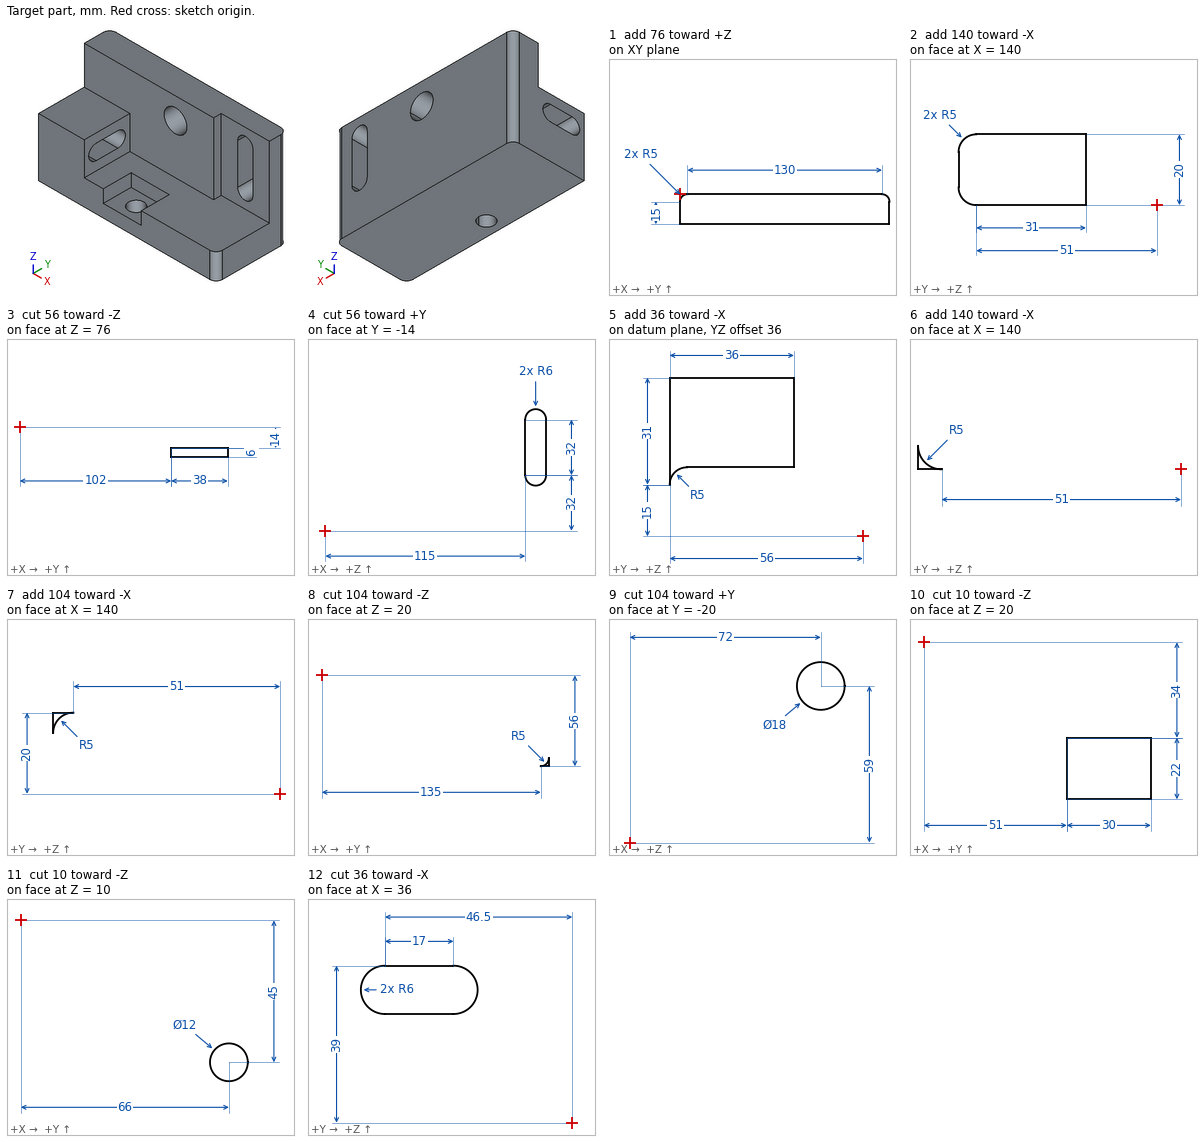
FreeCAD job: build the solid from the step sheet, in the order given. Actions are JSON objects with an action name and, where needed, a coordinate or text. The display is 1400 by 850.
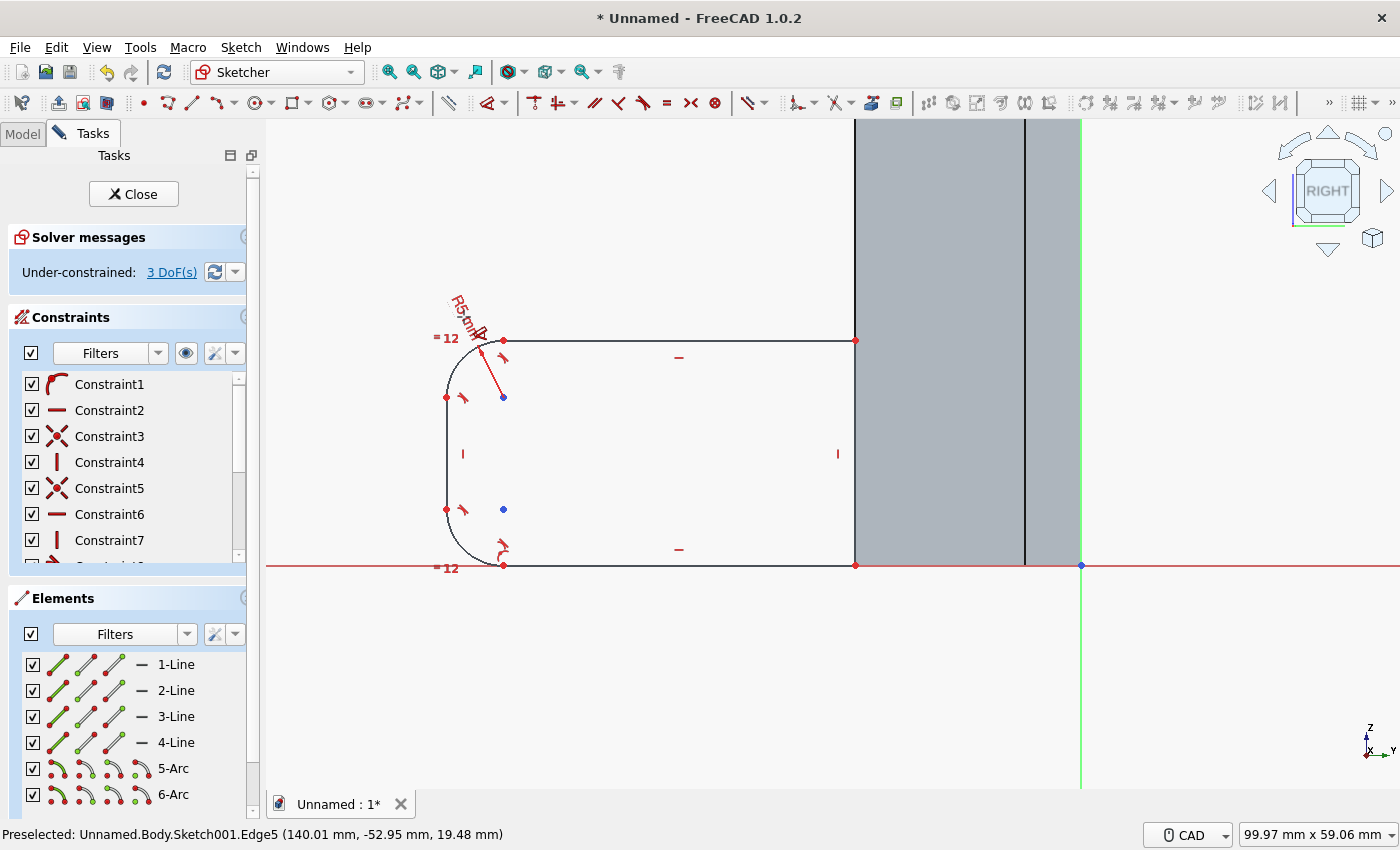
{"action": "left_click", "coordinate": [609, 566]}
{"action": "left_click", "coordinate": [679, 600]}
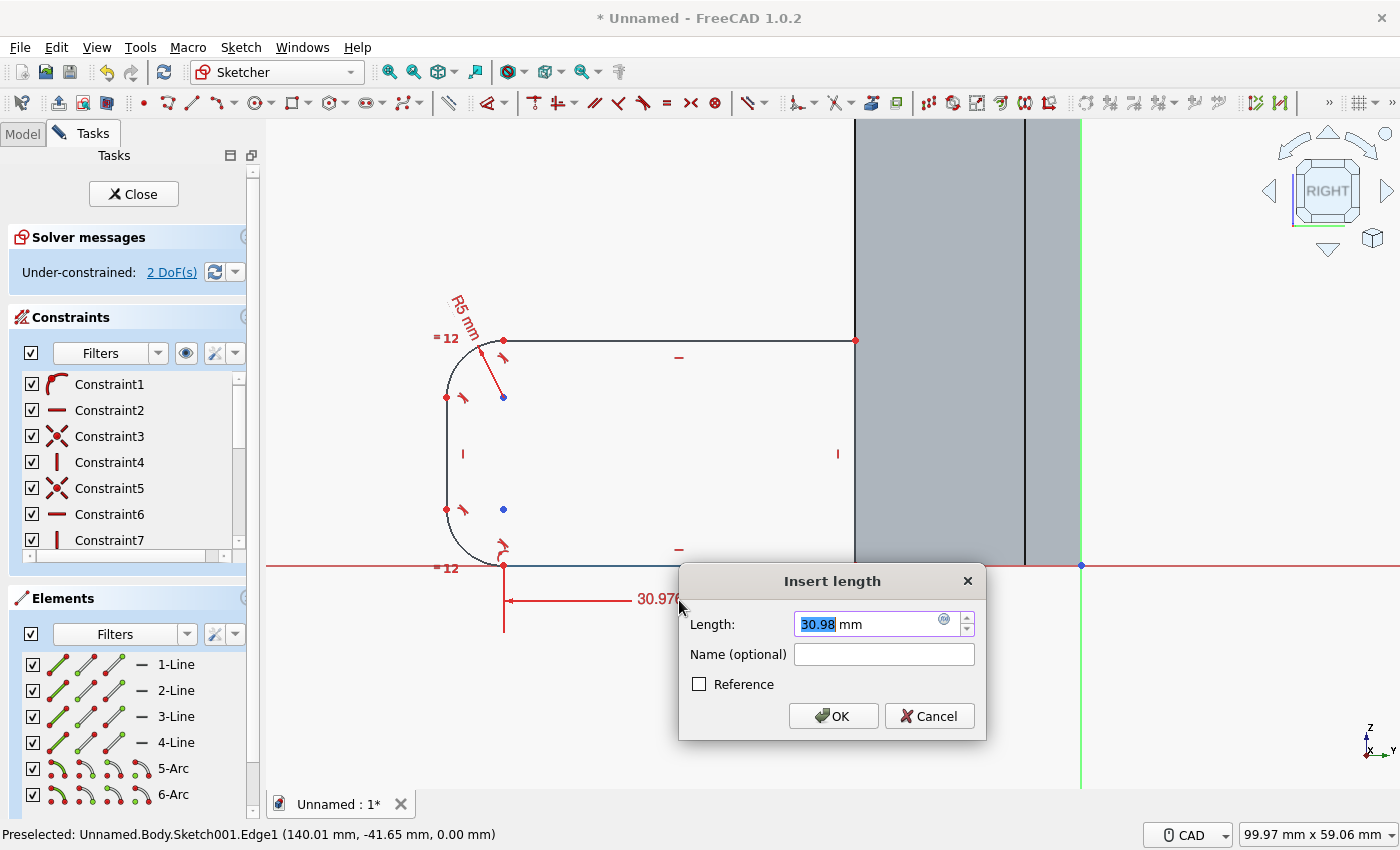
{"action": "type", "text": "31"}
{"action": "key", "text": "Return"}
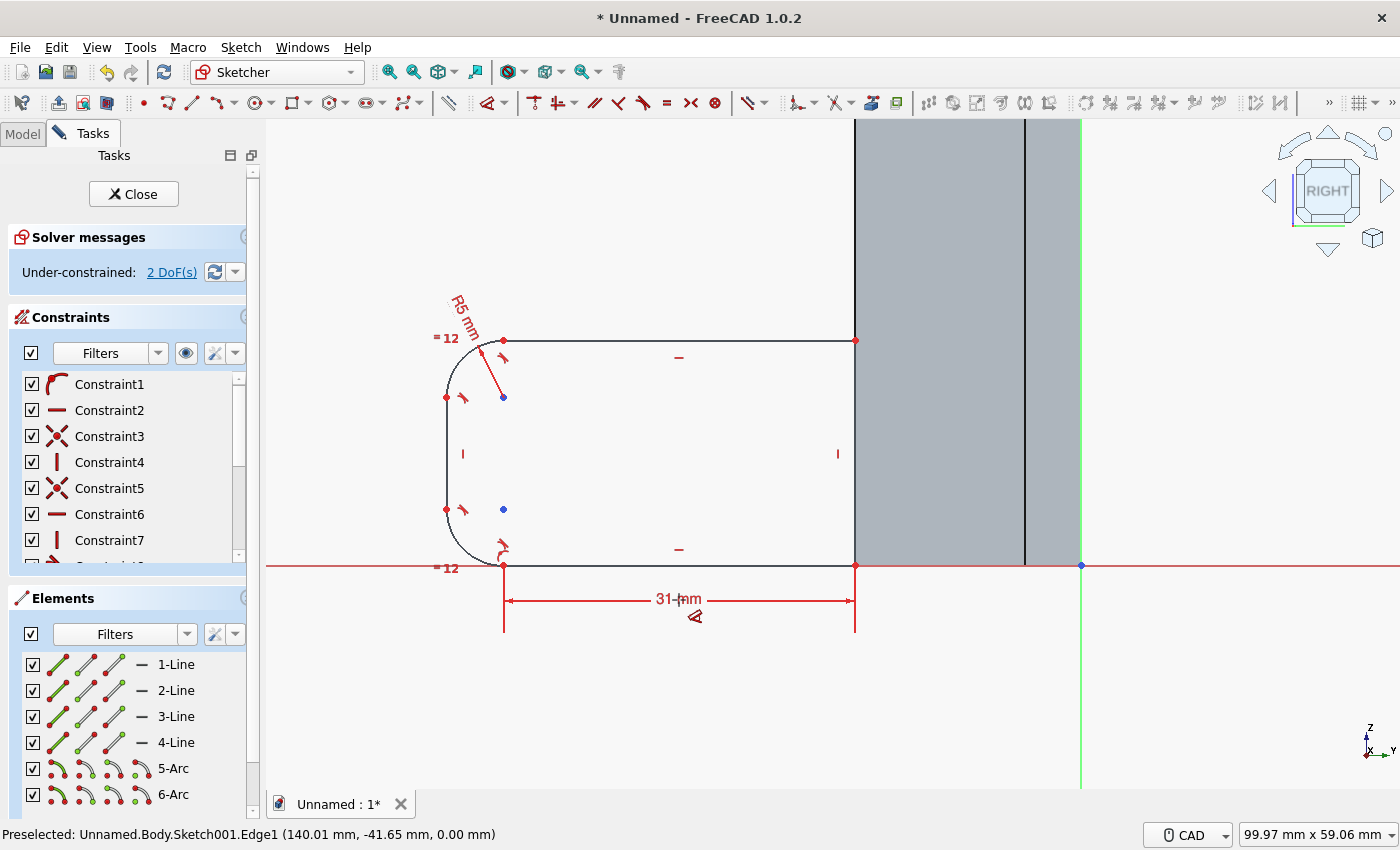
{"action": "left_click", "coordinate": [855, 498]}
{"action": "left_click", "coordinate": [889, 453]}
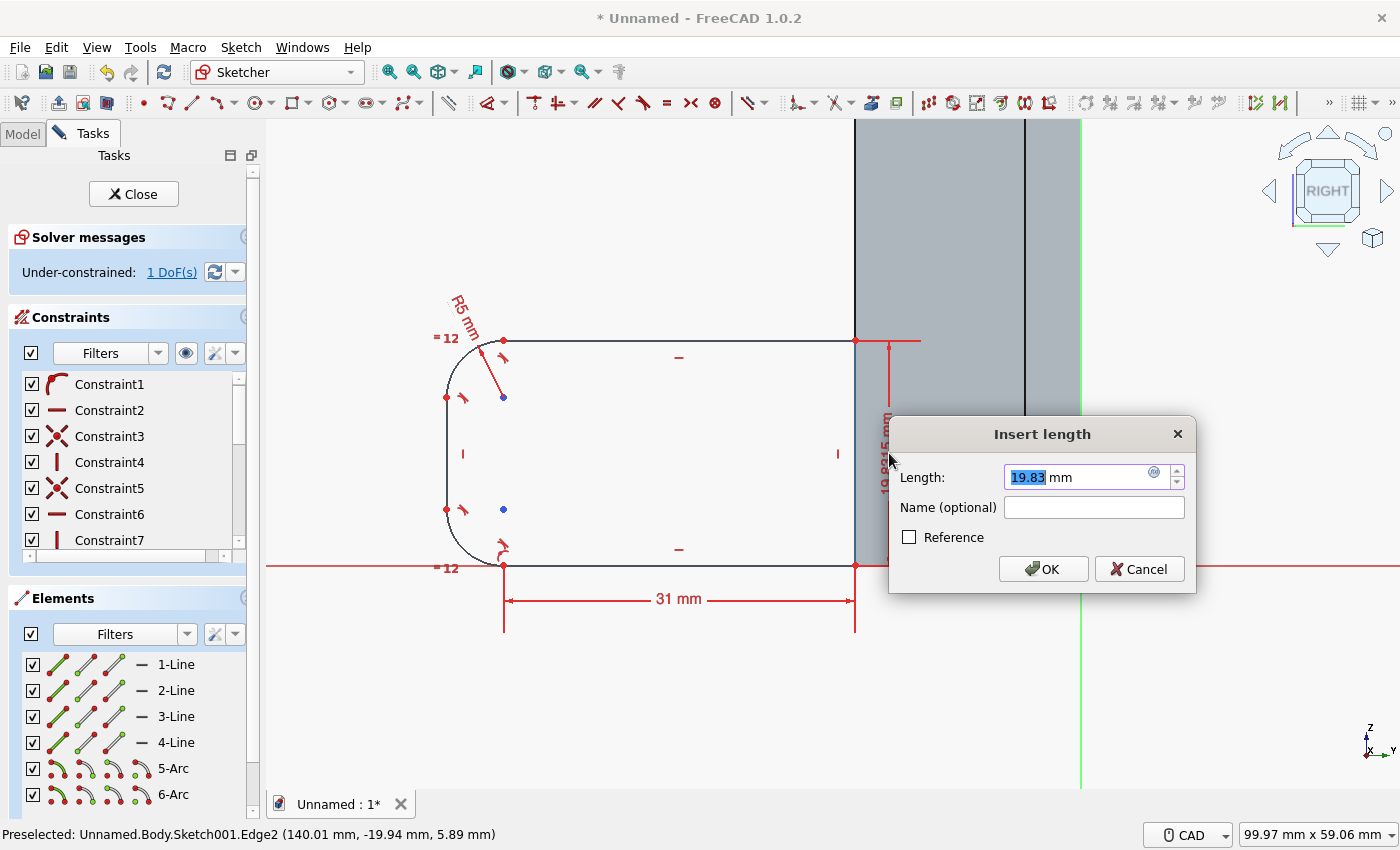
{"action": "type", "text": "20"}
{"action": "key", "text": "Return"}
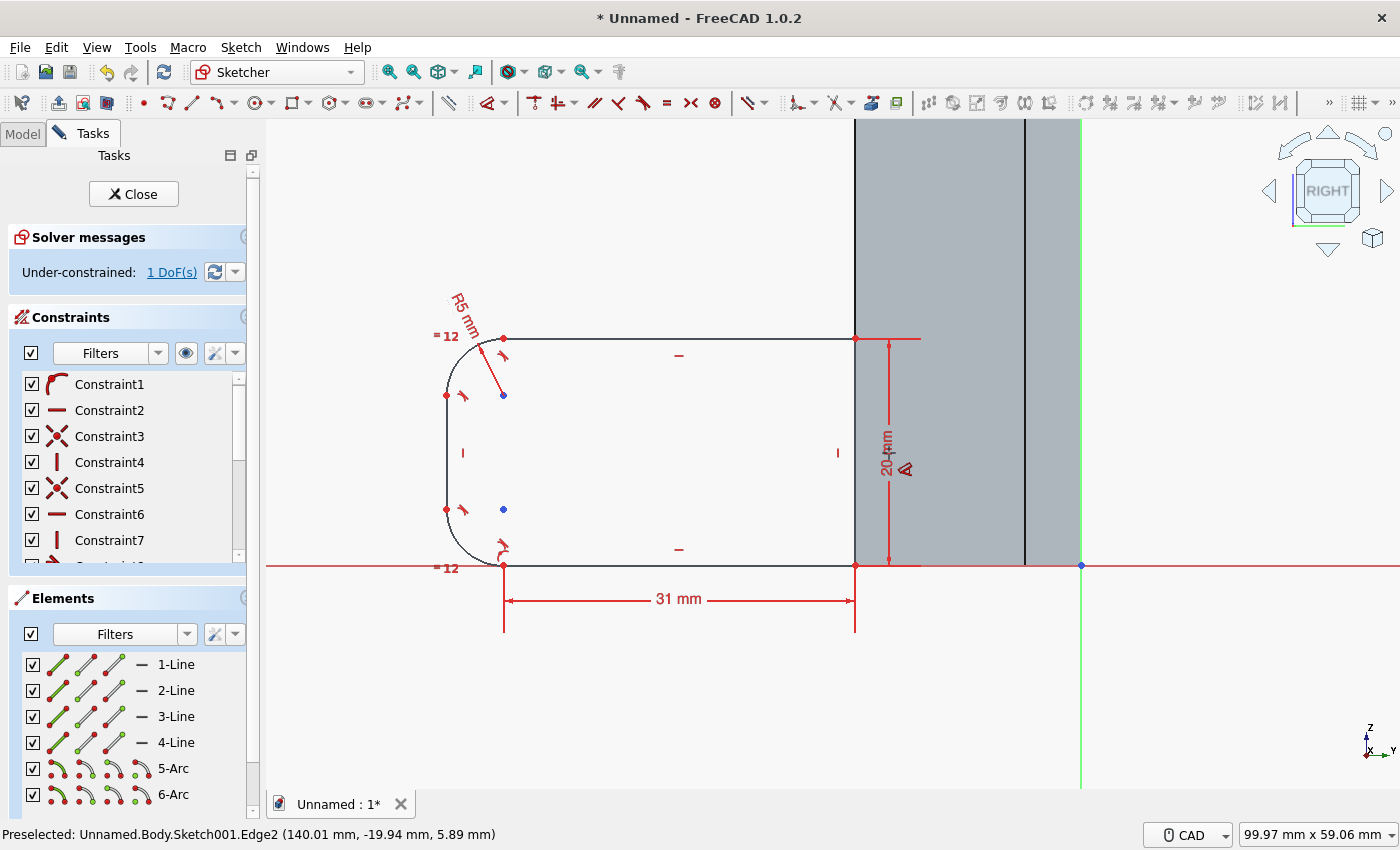
{"action": "left_click", "coordinate": [504, 566]}
{"action": "left_click", "coordinate": [793, 600]}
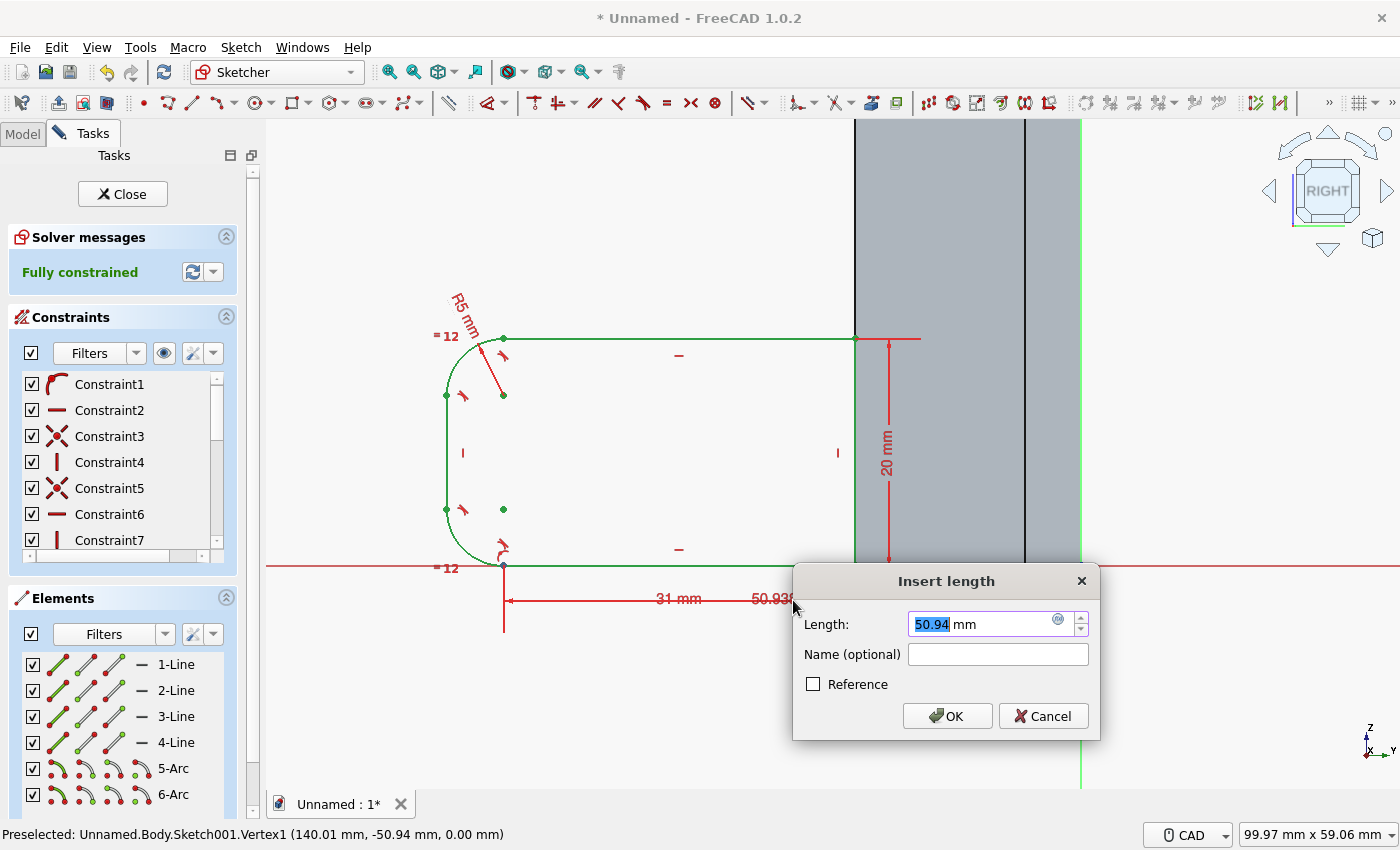
{"action": "type", "text": "51"}
{"action": "key", "text": "Return"}
{"action": "key", "text": "Escape"}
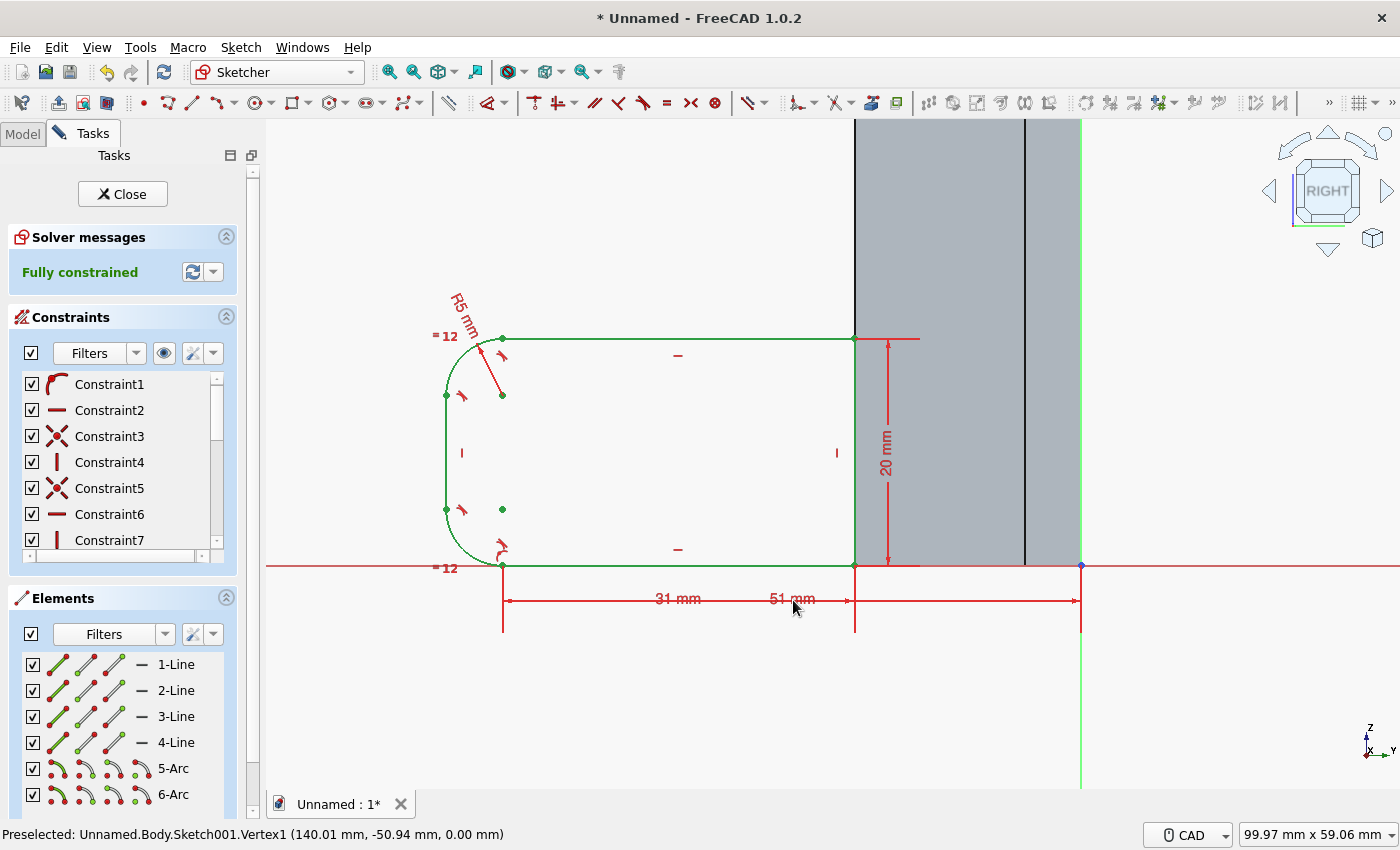
{"action": "left_click", "coordinate": [123, 194]}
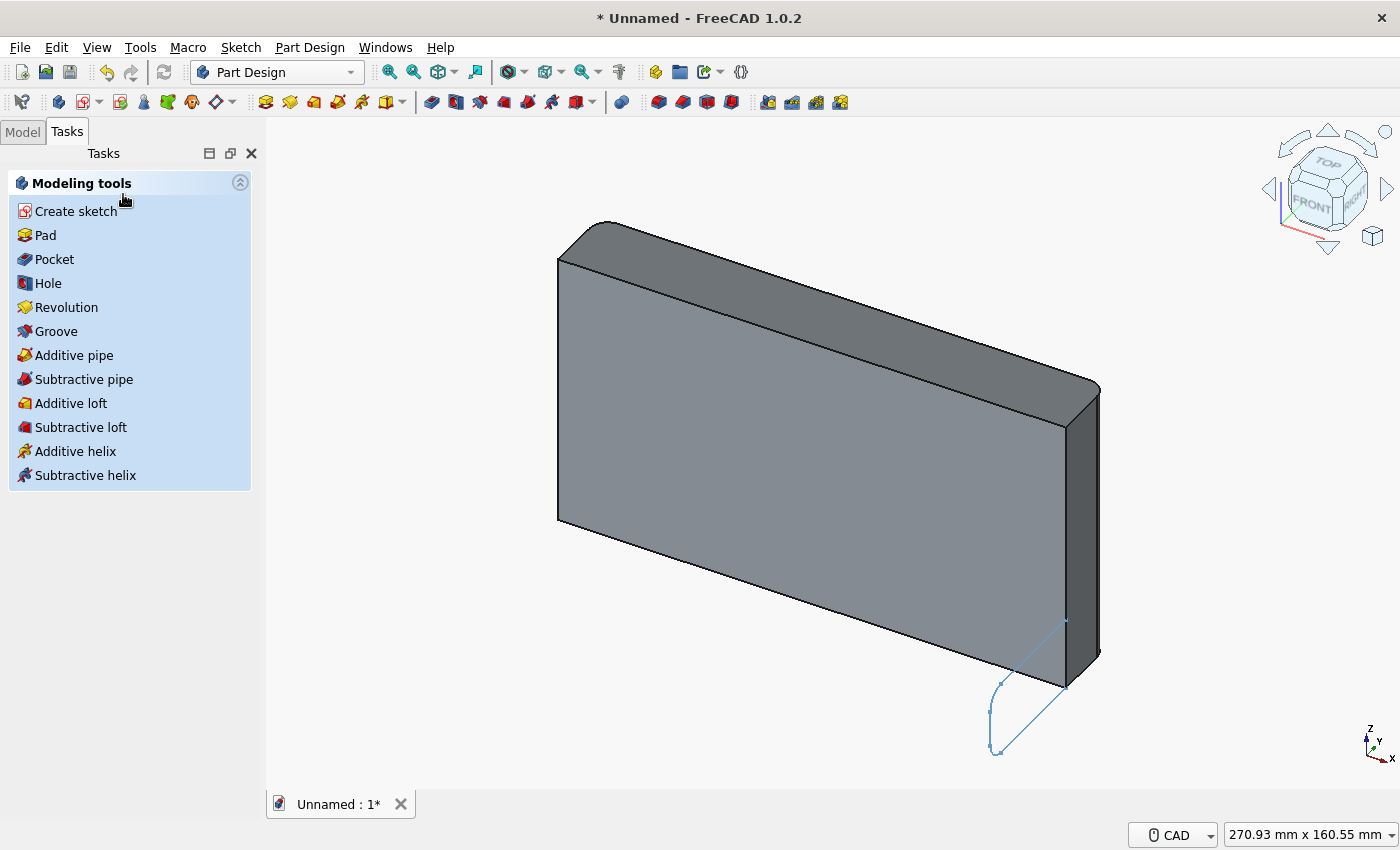
{"action": "left_click", "coordinate": [266, 102]}